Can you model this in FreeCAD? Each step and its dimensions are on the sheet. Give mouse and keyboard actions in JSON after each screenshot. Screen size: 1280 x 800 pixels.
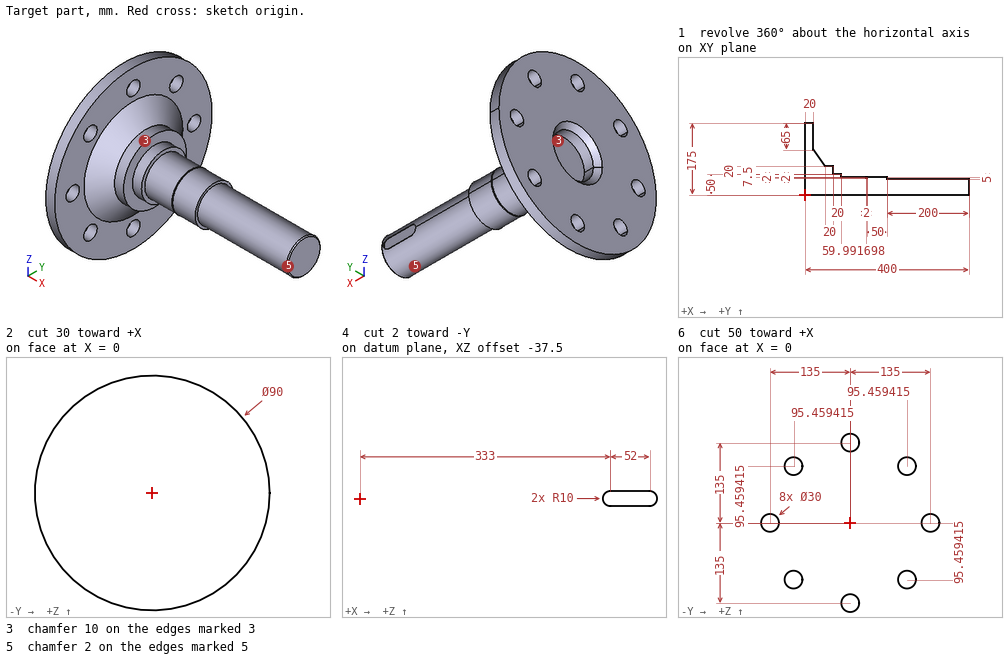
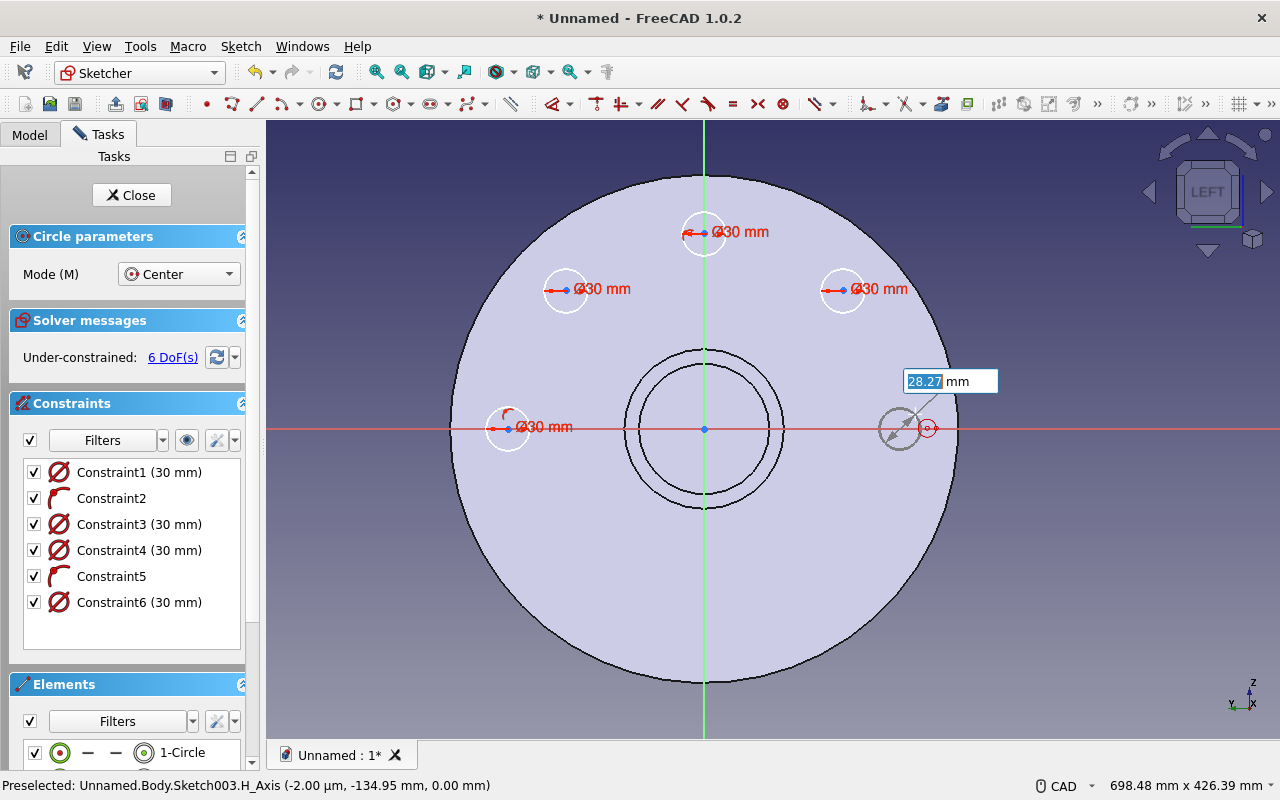
{"action": "type", "text": "30"}
{"action": "key", "text": "Return"}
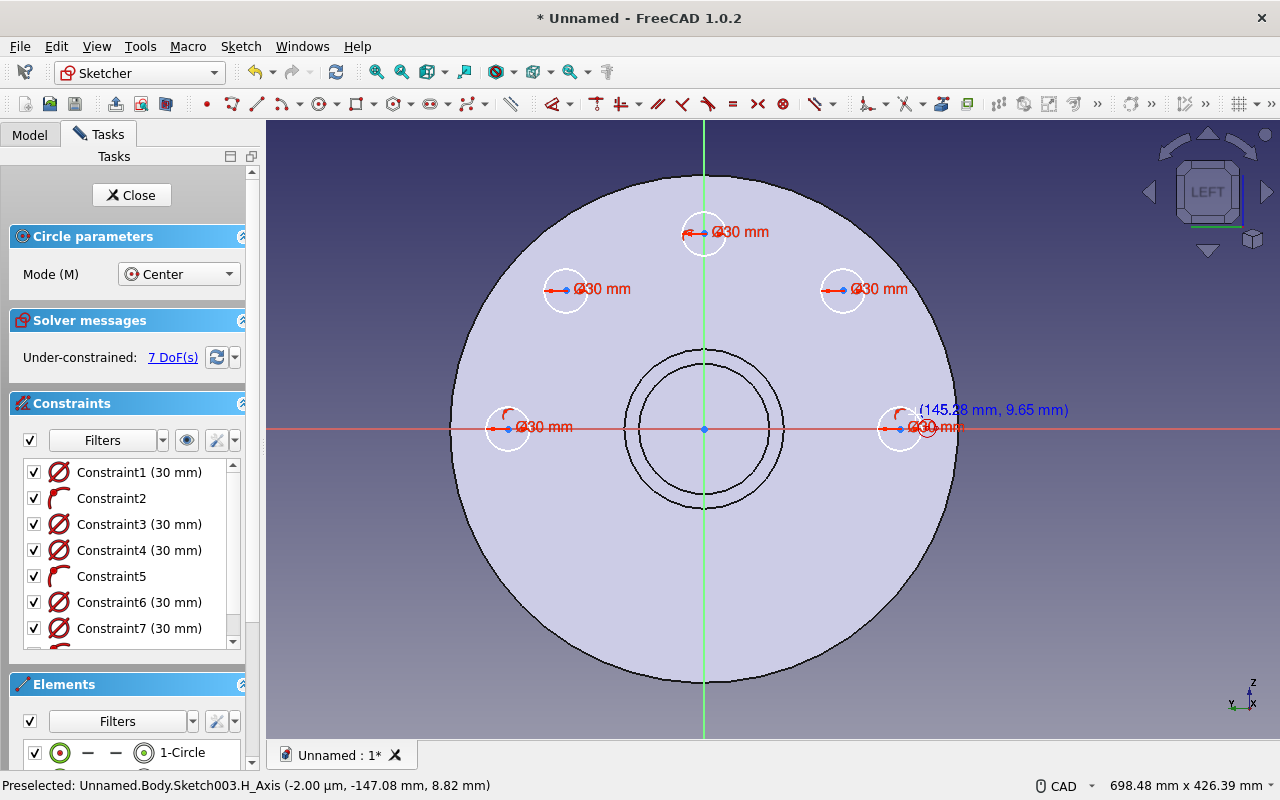
{"action": "left_click", "coordinate": [843, 568]}
{"action": "mouse_move", "coordinate": [858, 552]}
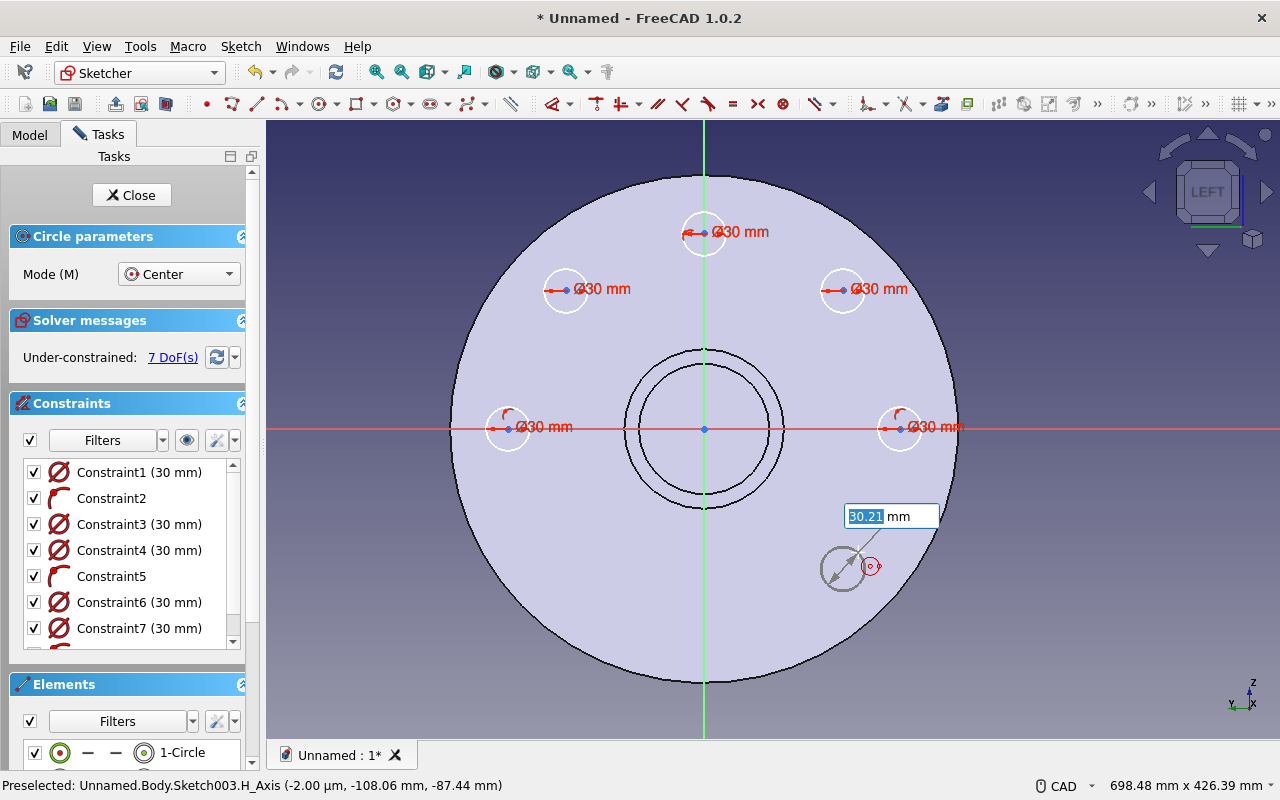
{"action": "type", "text": "30"}
{"action": "key", "text": "Return"}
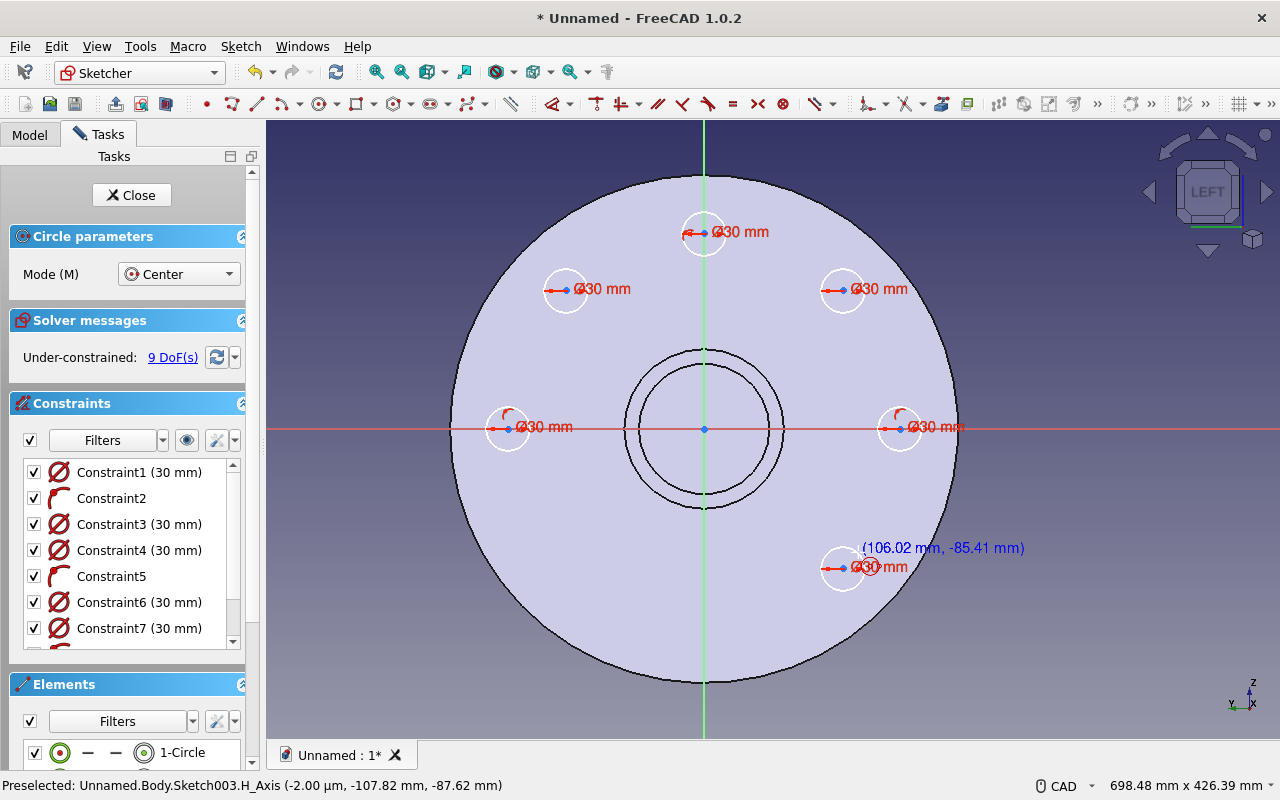
{"action": "left_click", "coordinate": [704, 625]}
{"action": "mouse_move", "coordinate": [719, 610]}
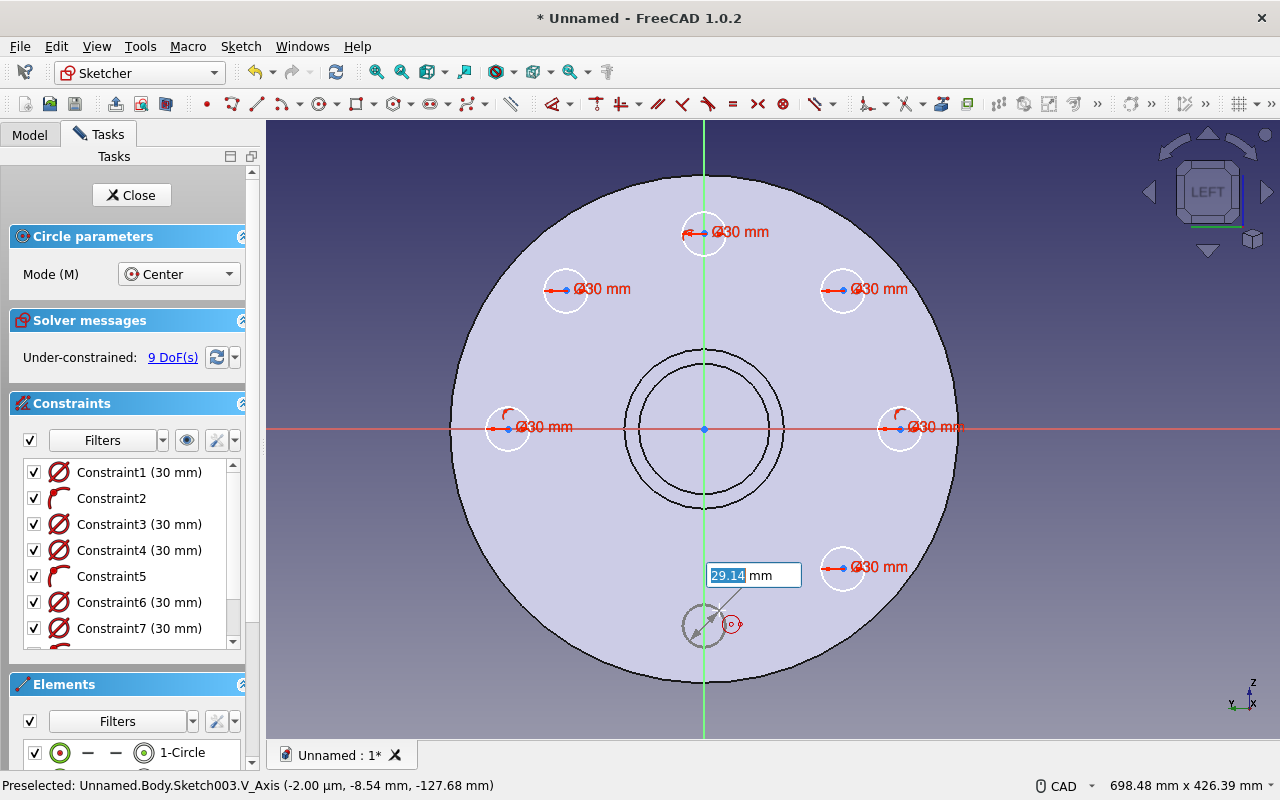
{"action": "type", "text": "30"}
{"action": "key", "text": "Return"}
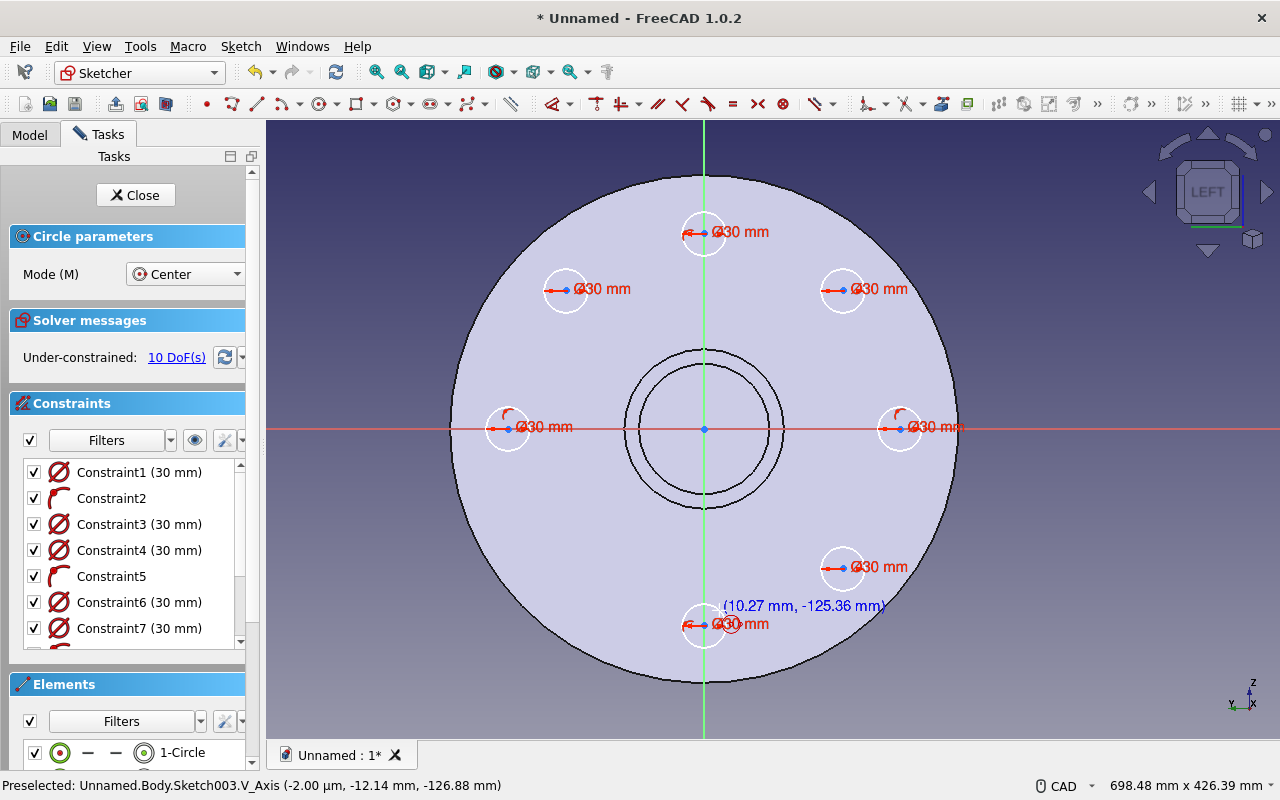
{"action": "left_click", "coordinate": [566, 568]}
{"action": "mouse_move", "coordinate": [581, 552]}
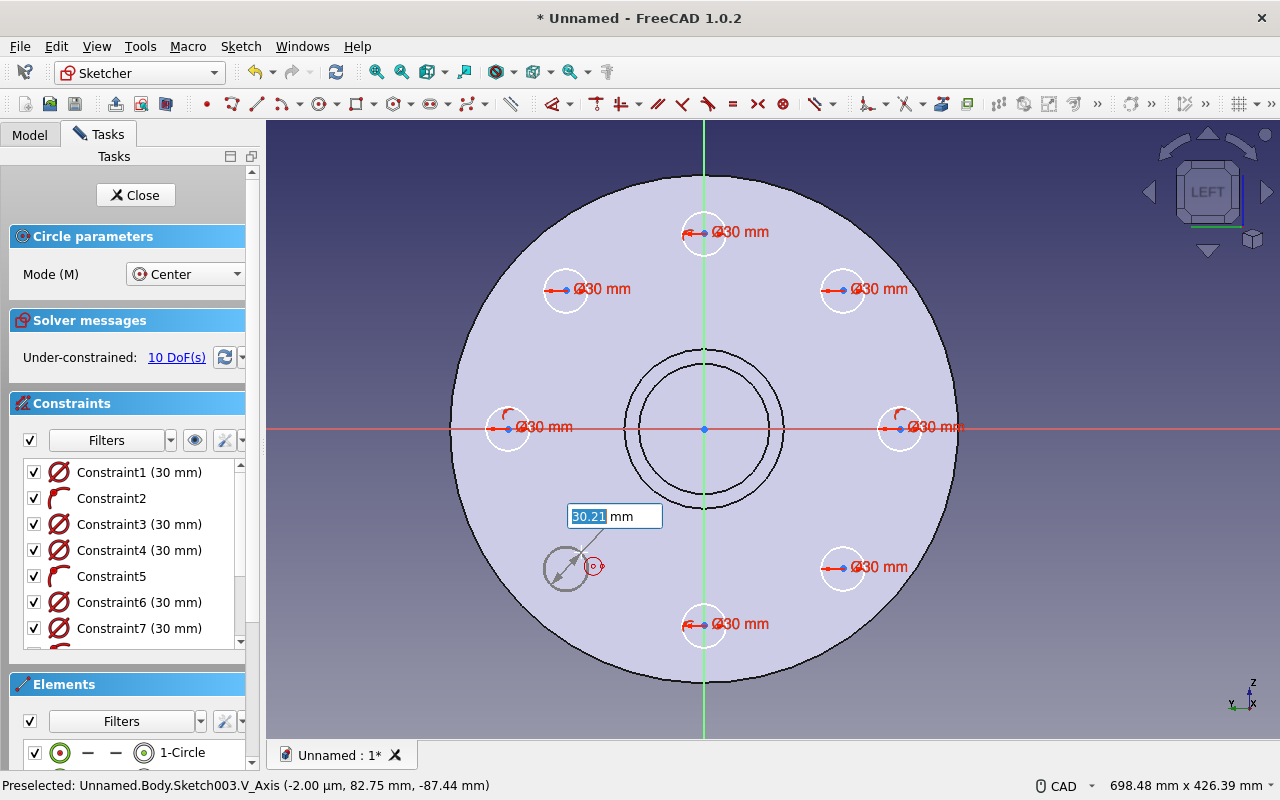
{"action": "type", "text": "30"}
{"action": "key", "text": "Return"}
{"action": "key", "text": "Escape"}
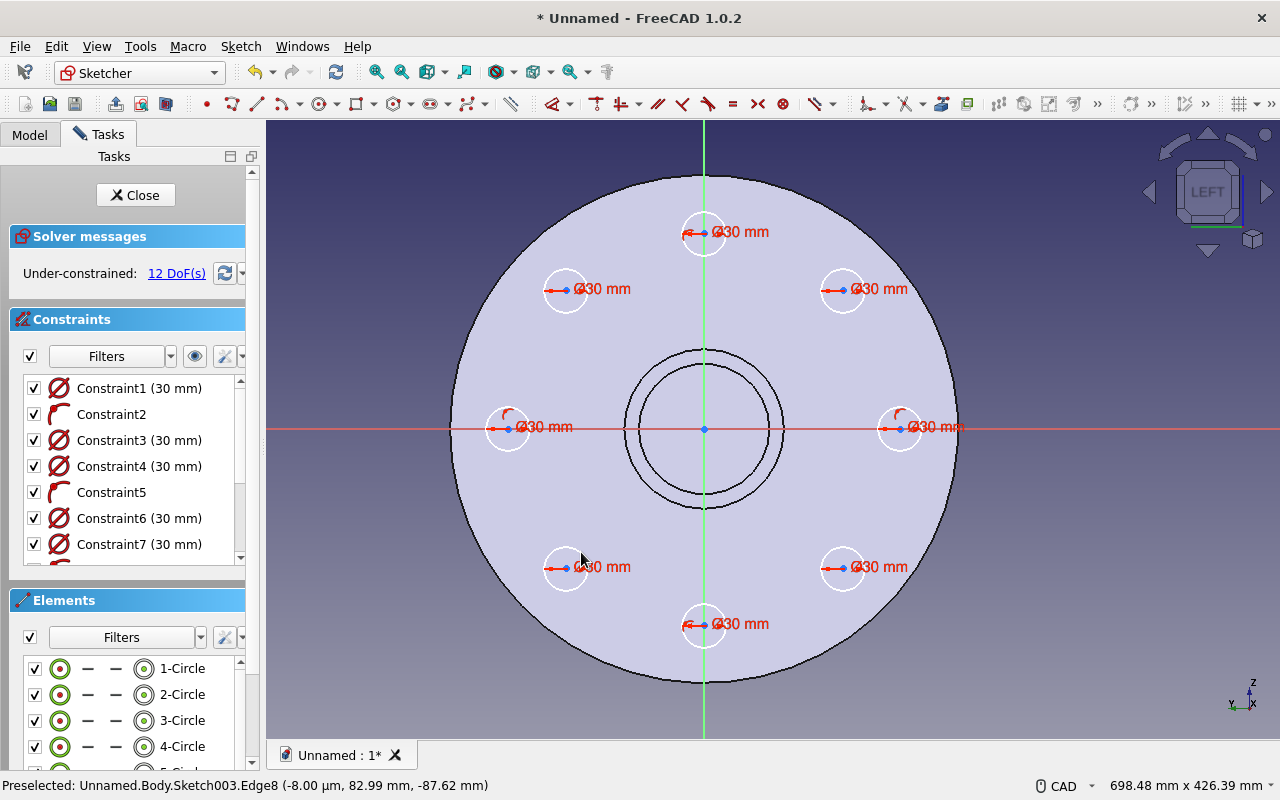
{"action": "left_click", "coordinate": [566, 291]}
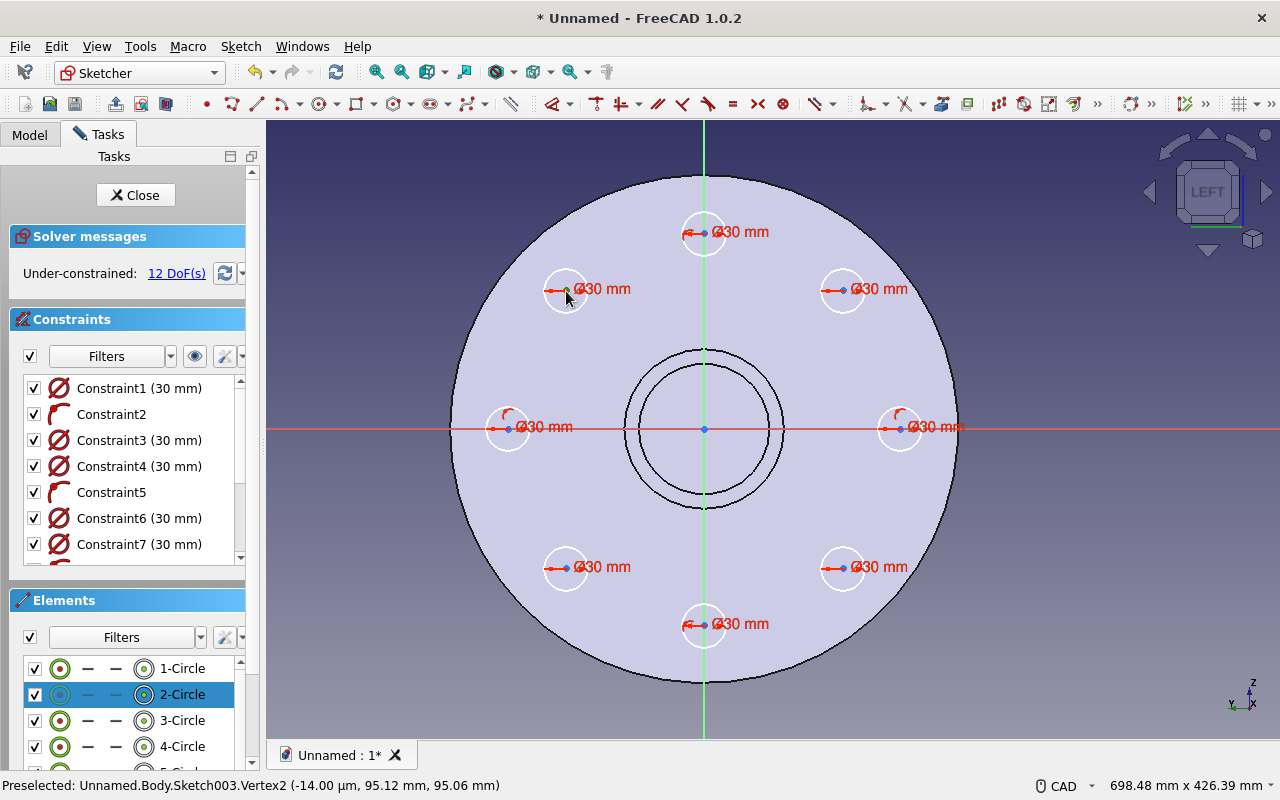
{"action": "left_click", "coordinate": [843, 291]}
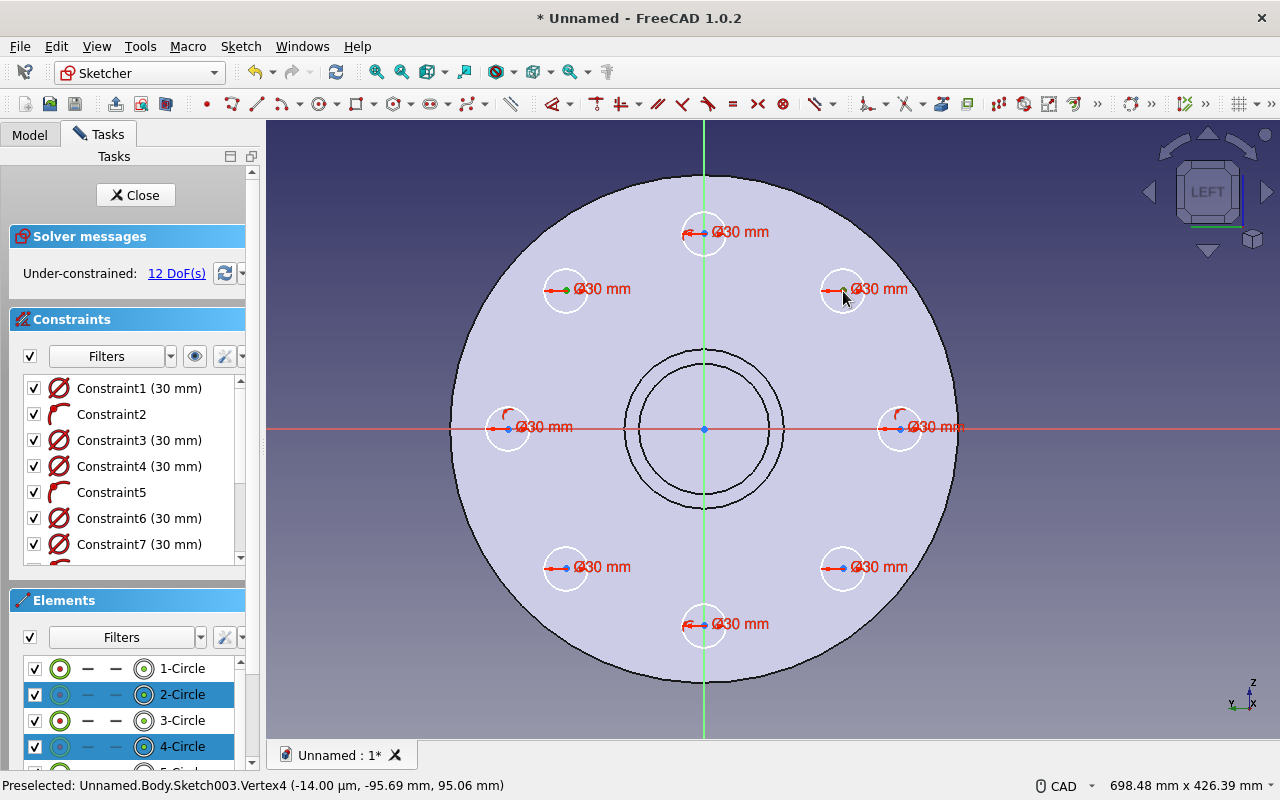
{"action": "key", "text": "h"}